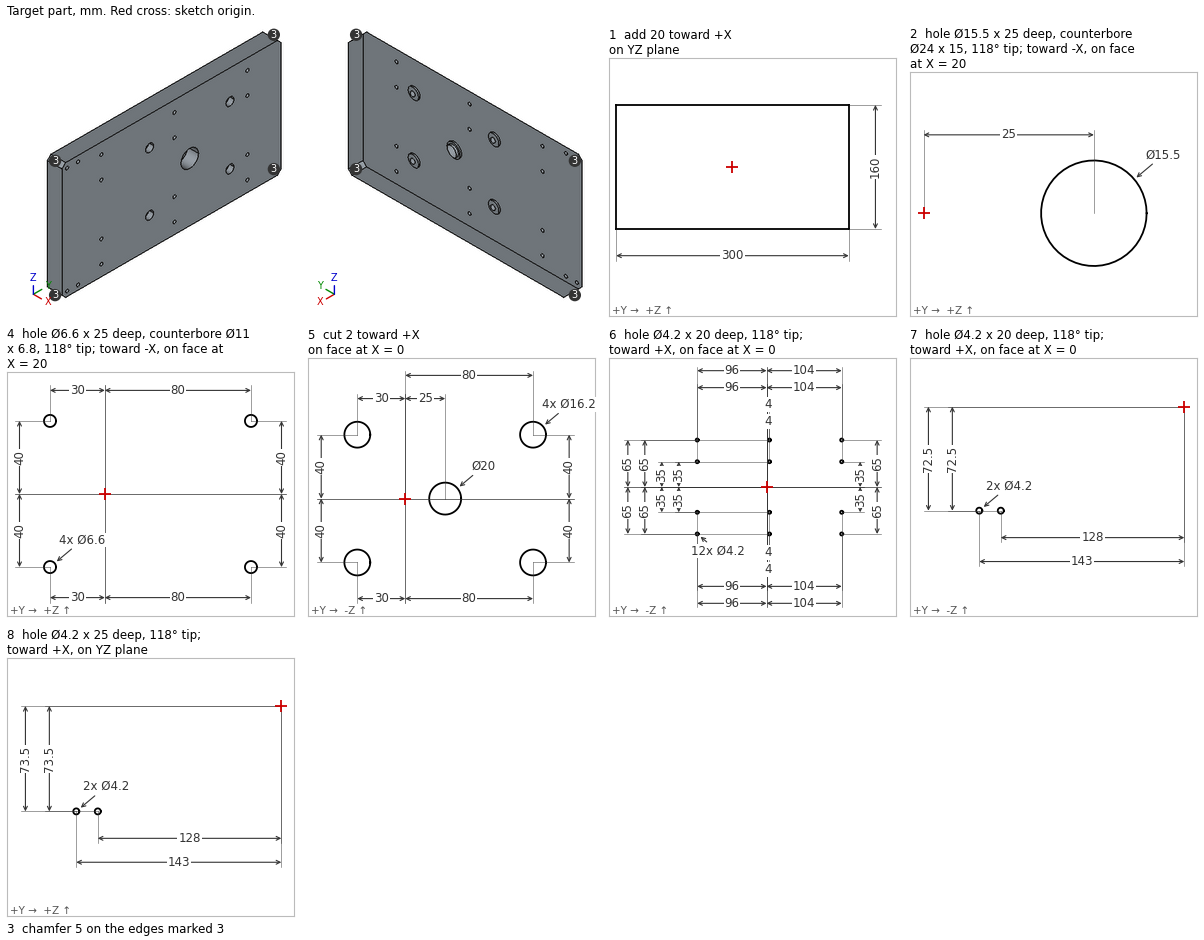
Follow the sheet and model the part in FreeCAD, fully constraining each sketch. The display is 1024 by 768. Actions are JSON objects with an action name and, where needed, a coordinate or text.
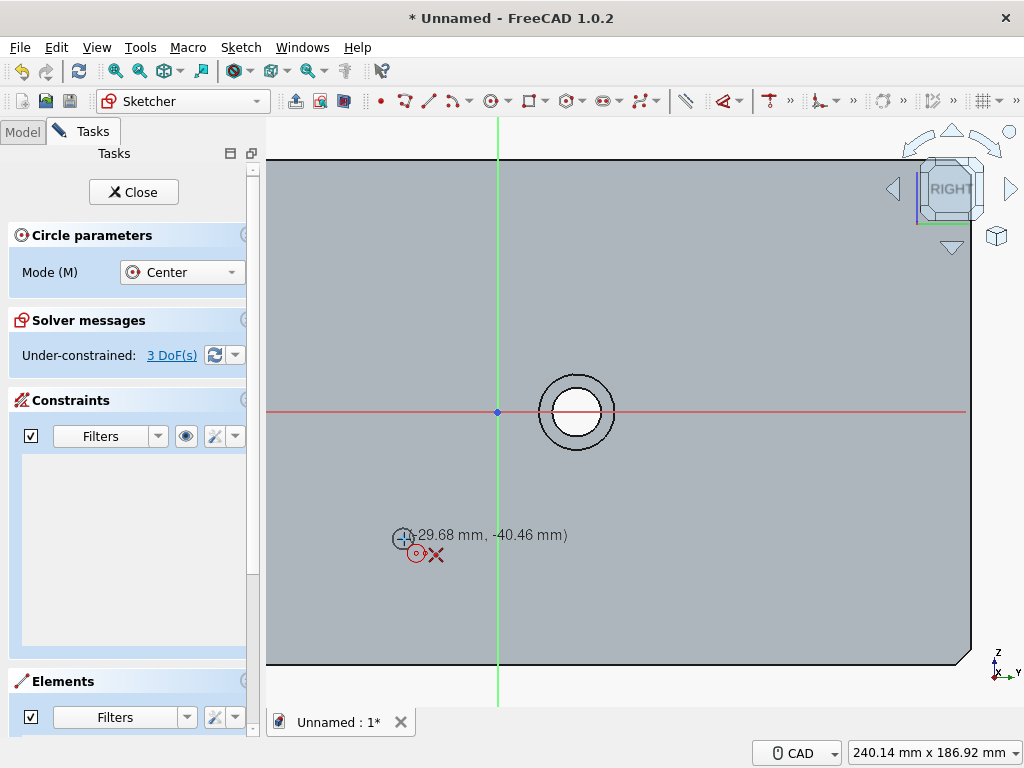
{"action": "scroll", "coordinate": [750, 538], "scroll_direction": "up", "scroll_amount": 4}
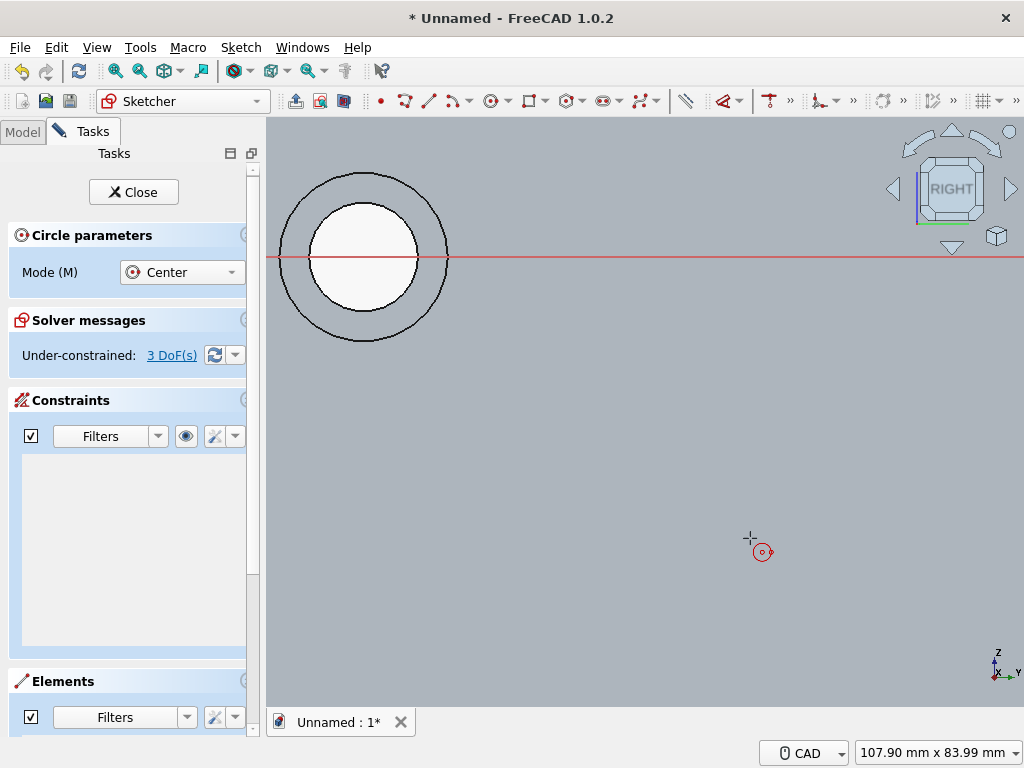
{"action": "left_click", "coordinate": [750, 538]}
{"action": "left_click", "coordinate": [766, 522]}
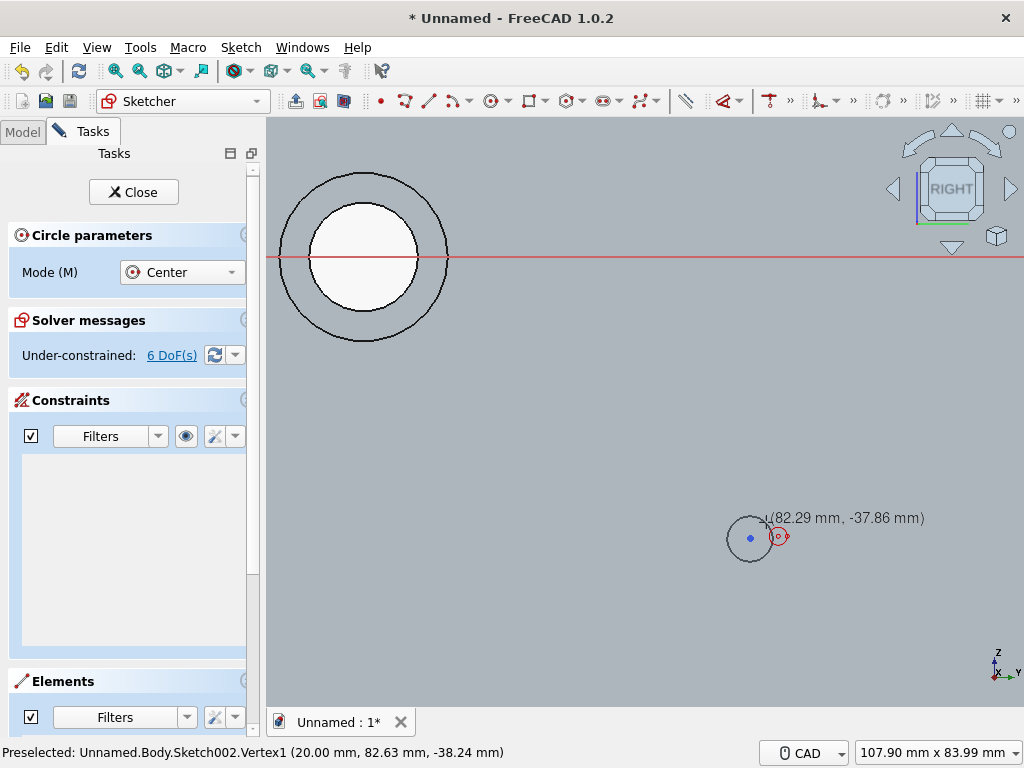
{"action": "scroll", "coordinate": [750, 538], "scroll_direction": "down", "scroll_amount": 4}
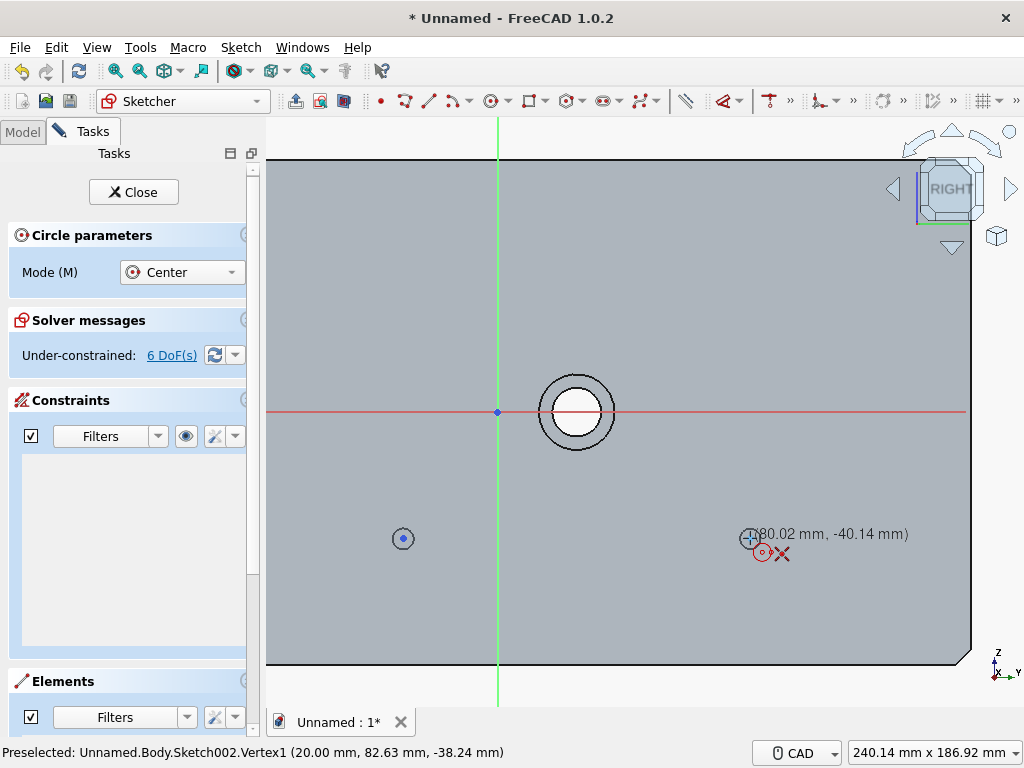
{"action": "scroll", "coordinate": [403, 286], "scroll_direction": "up", "scroll_amount": 4}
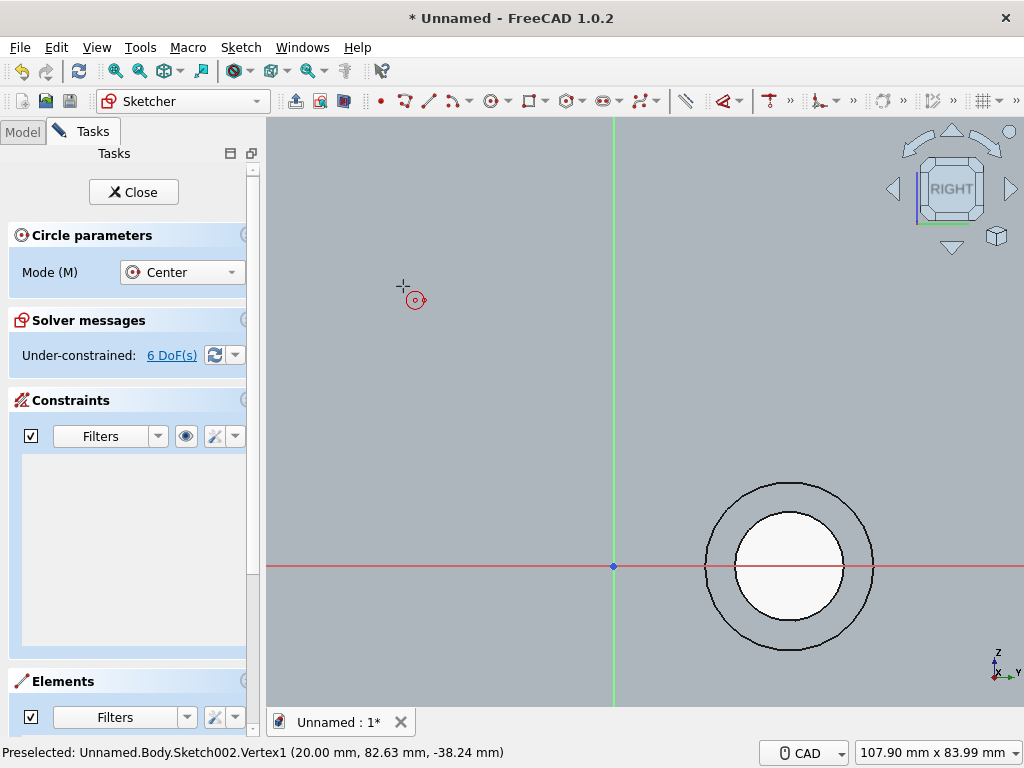
{"action": "left_click", "coordinate": [403, 285]}
{"action": "left_click", "coordinate": [419, 269]}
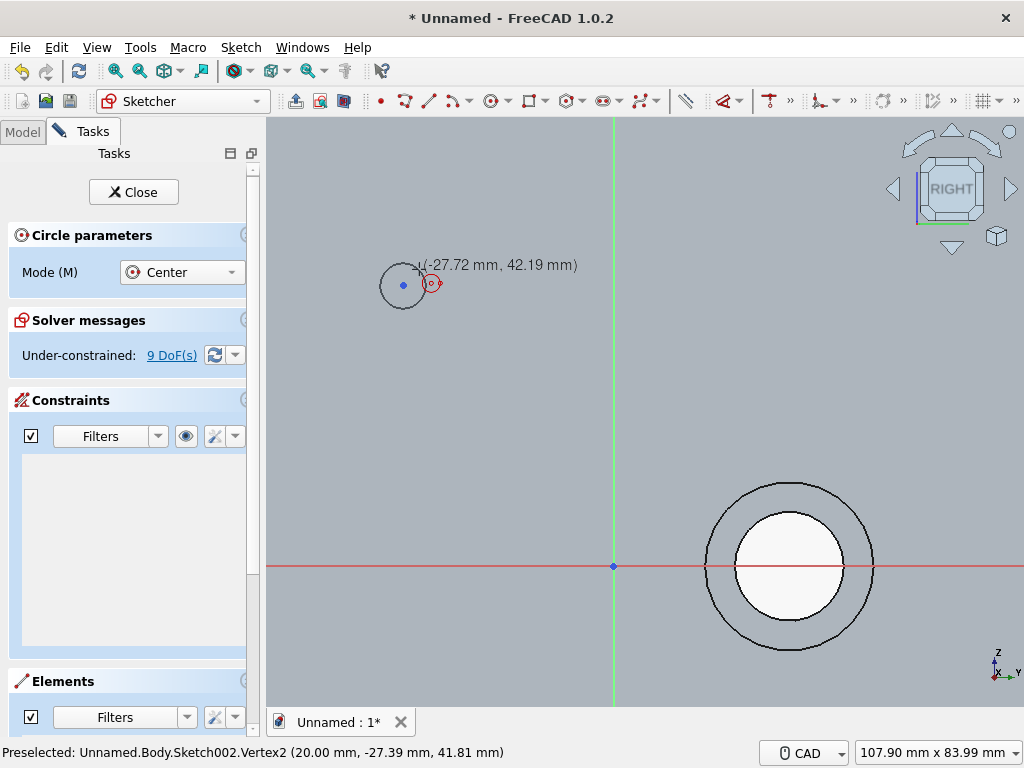
{"action": "scroll", "coordinate": [403, 286], "scroll_direction": "down", "scroll_amount": 4}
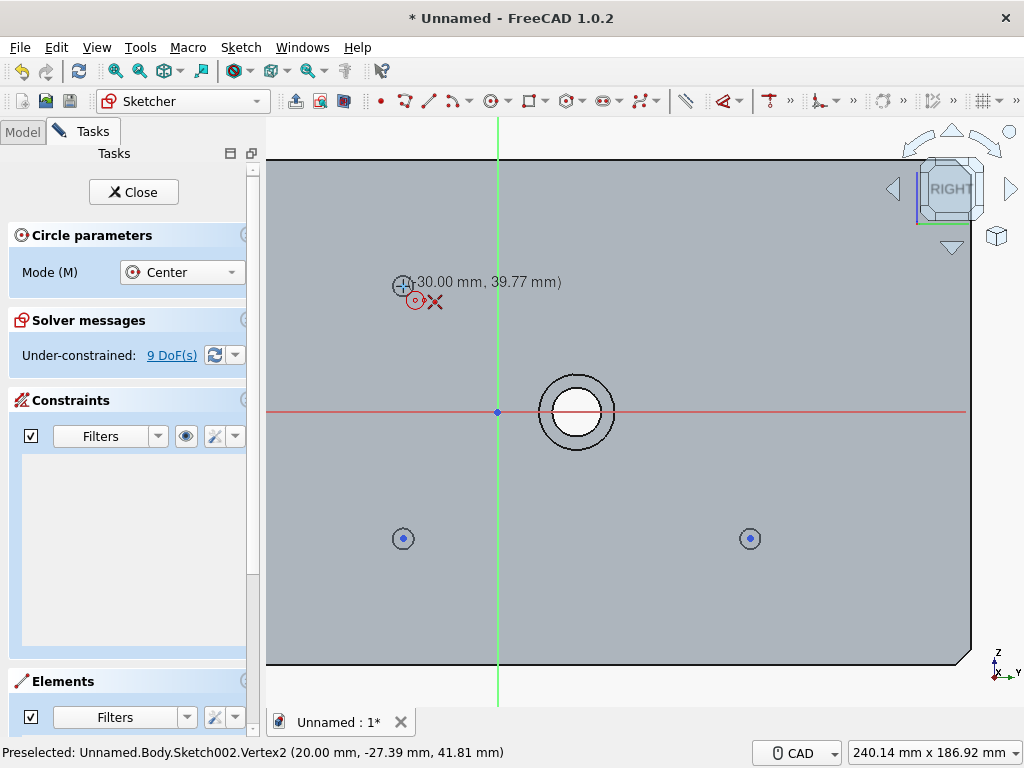
{"action": "scroll", "coordinate": [750, 286], "scroll_direction": "up", "scroll_amount": 4}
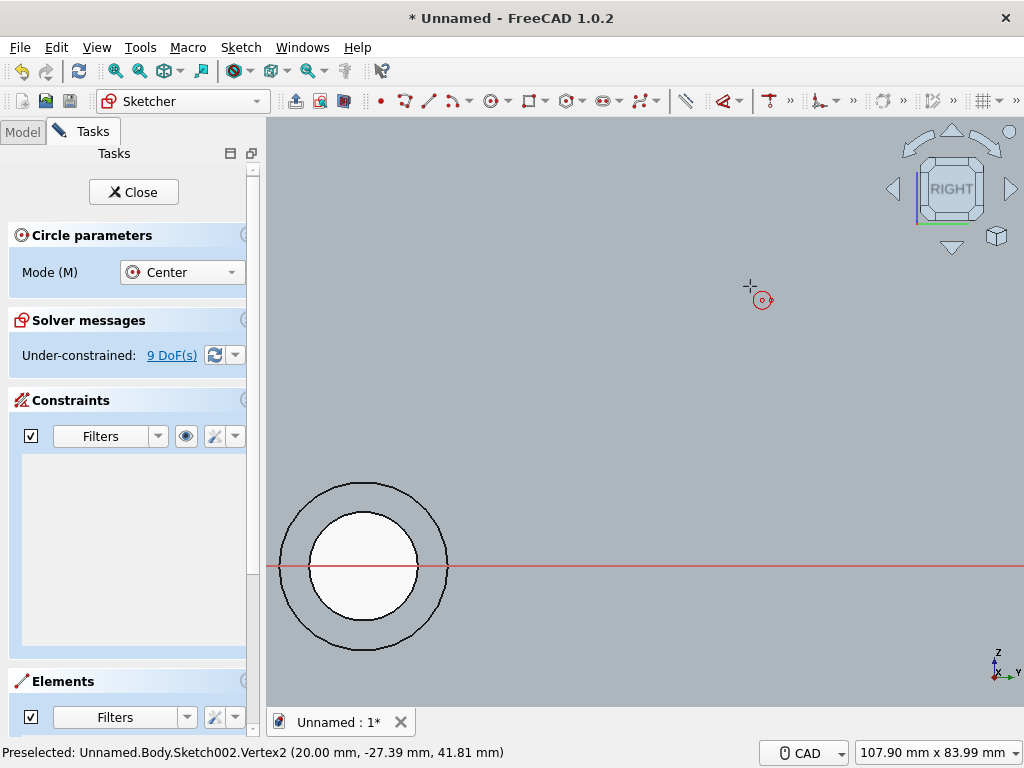
{"action": "left_click", "coordinate": [750, 285]}
{"action": "left_click", "coordinate": [766, 269]}
{"action": "key", "text": "Escape"}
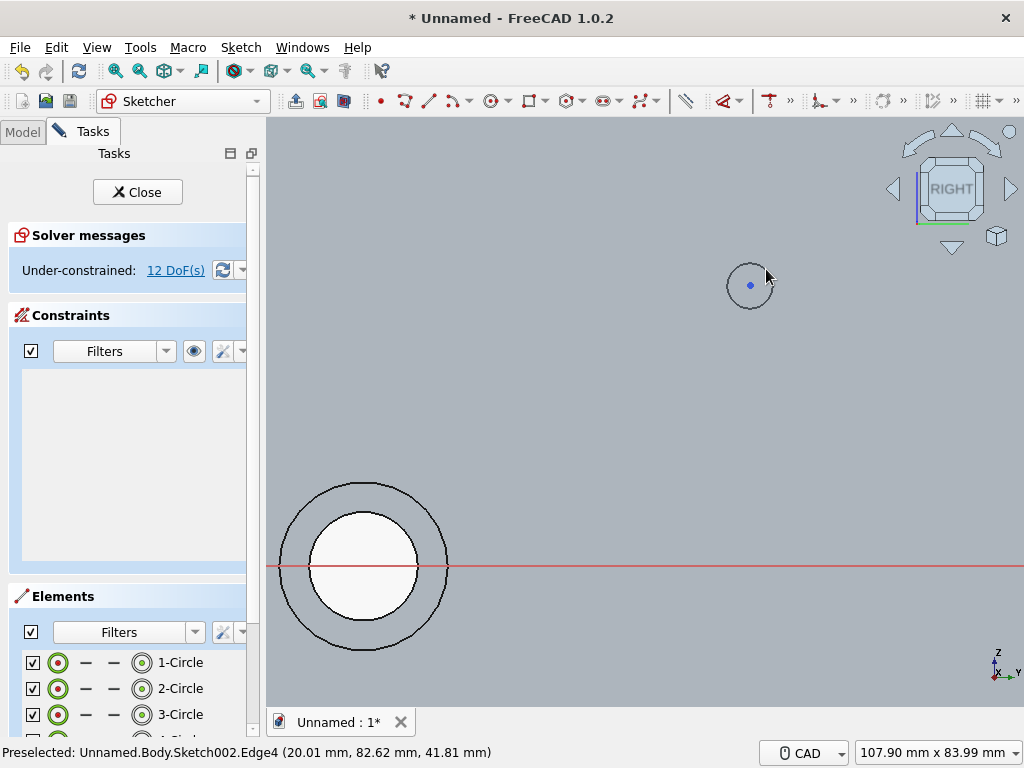
{"action": "scroll", "coordinate": [750, 286], "scroll_direction": "down", "scroll_amount": 4}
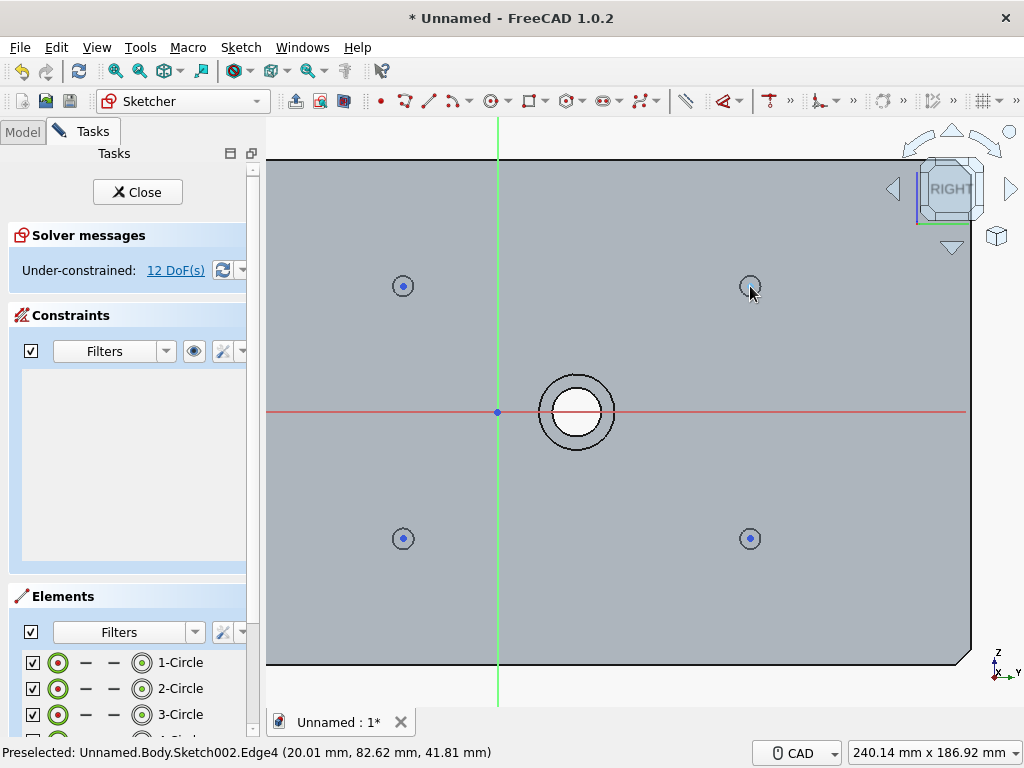
{"action": "scroll", "coordinate": [411, 532], "scroll_direction": "up", "scroll_amount": 2}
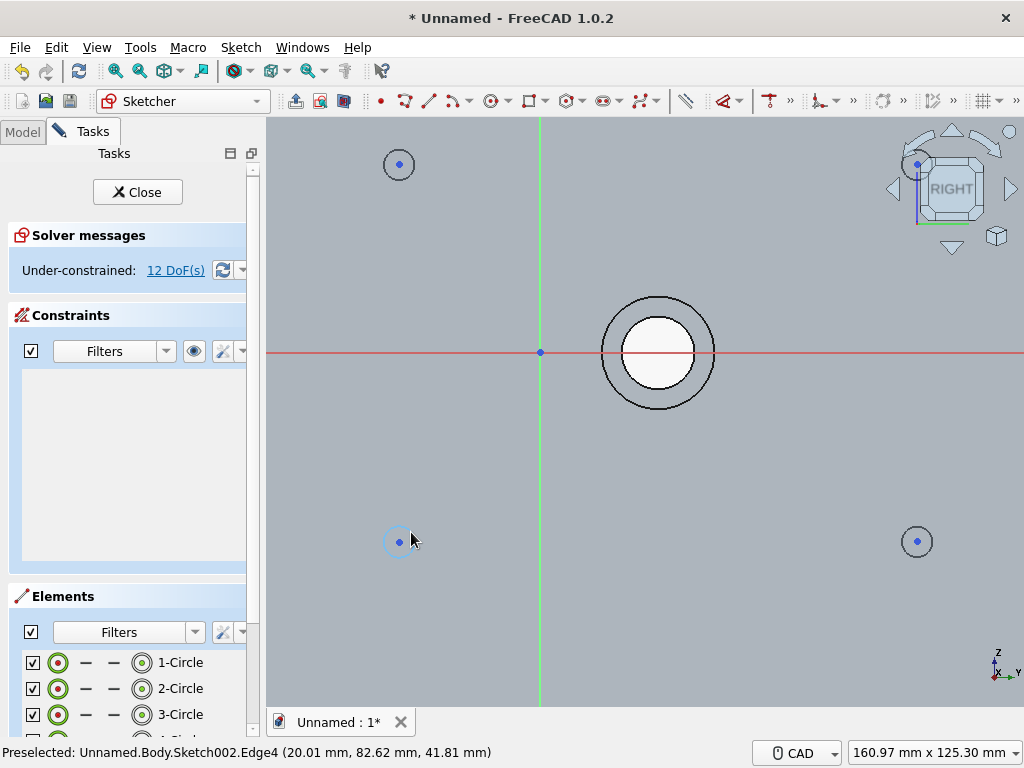
{"action": "left_click", "coordinate": [410, 531]}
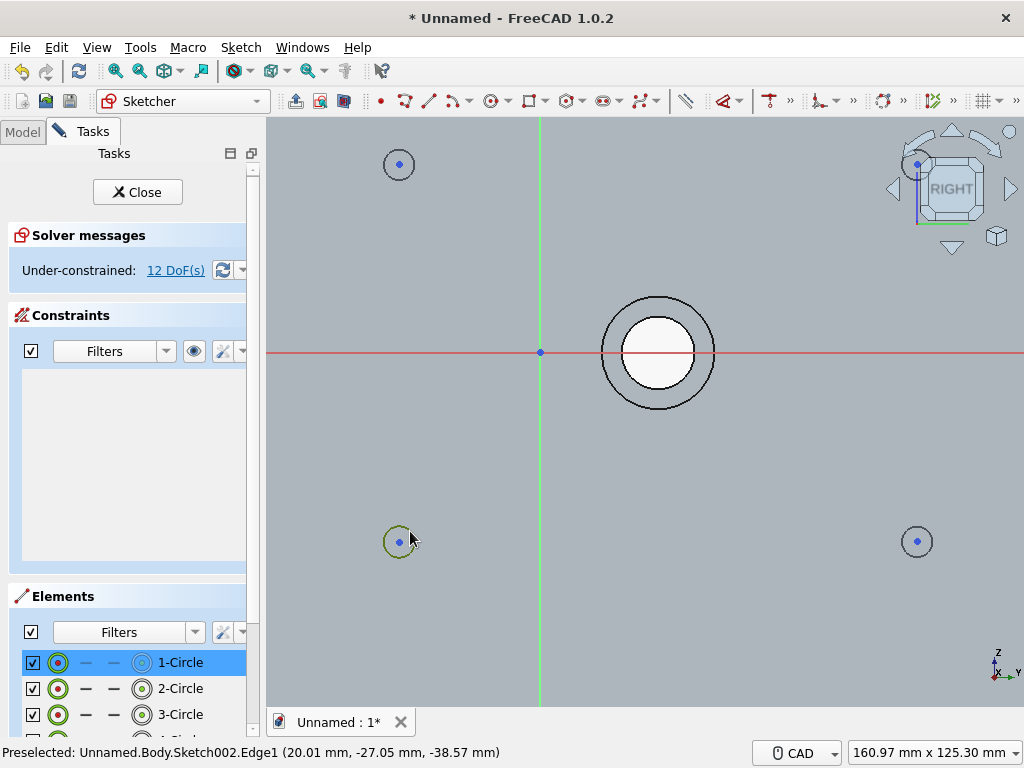
{"action": "scroll", "coordinate": [411, 532], "scroll_direction": "down", "scroll_amount": 2}